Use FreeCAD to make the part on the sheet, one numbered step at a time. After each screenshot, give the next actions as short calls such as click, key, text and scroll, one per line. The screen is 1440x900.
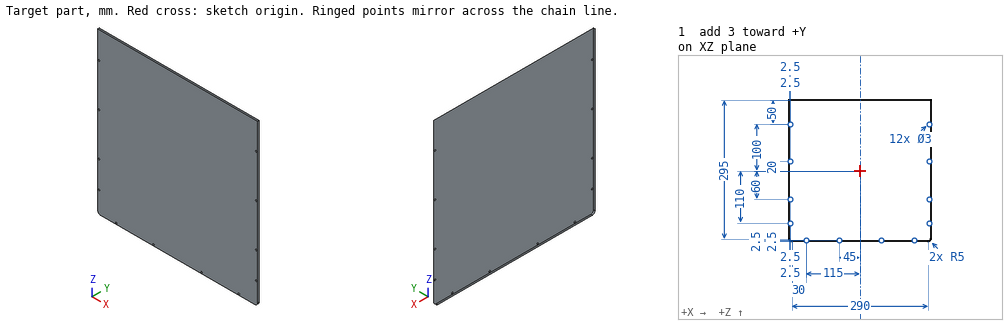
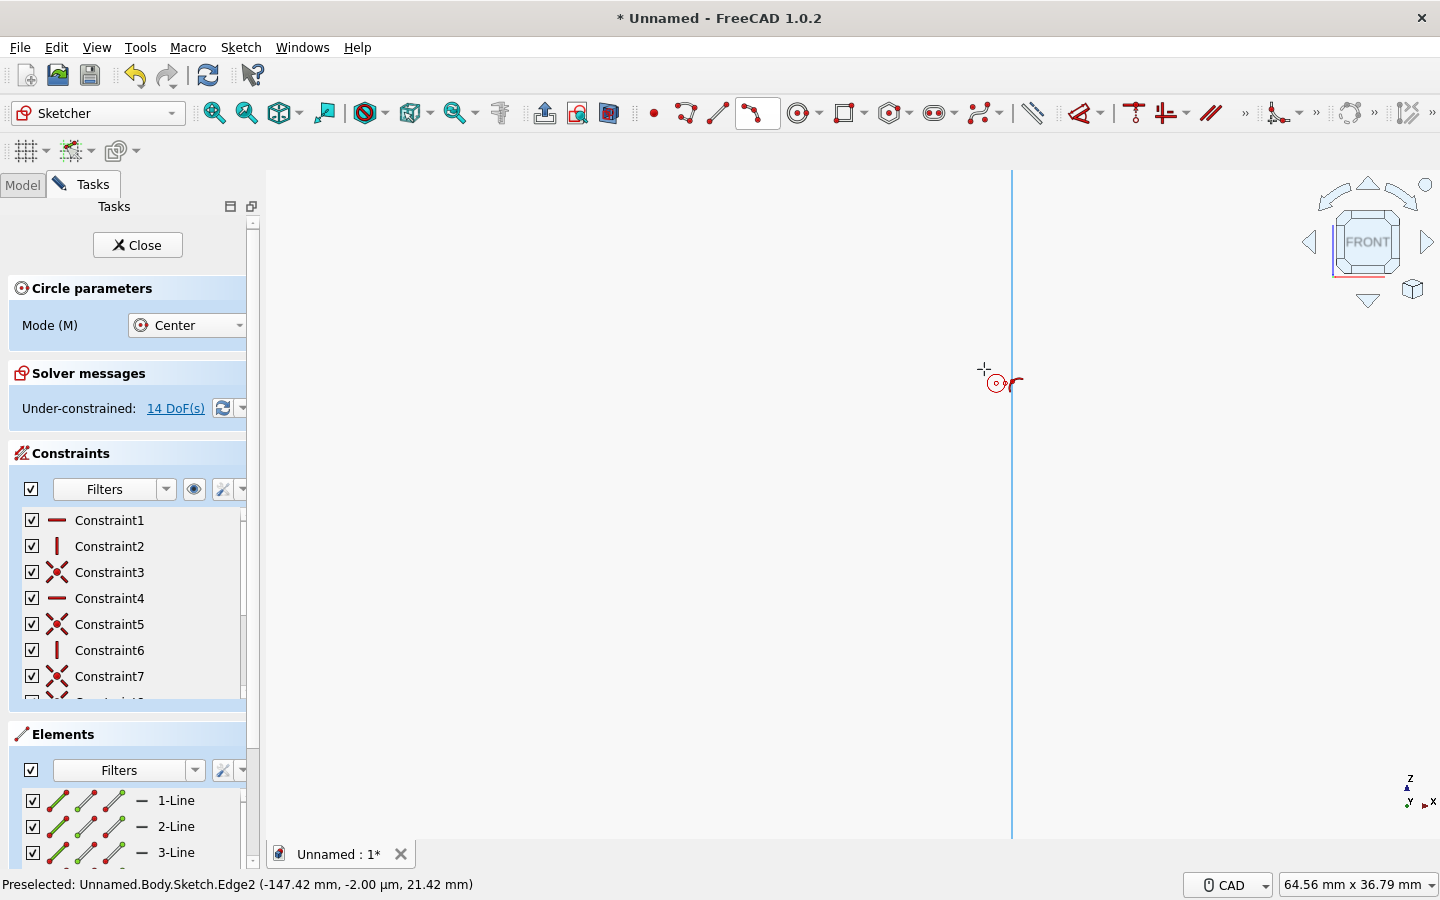
click(971, 371)
move(990, 352)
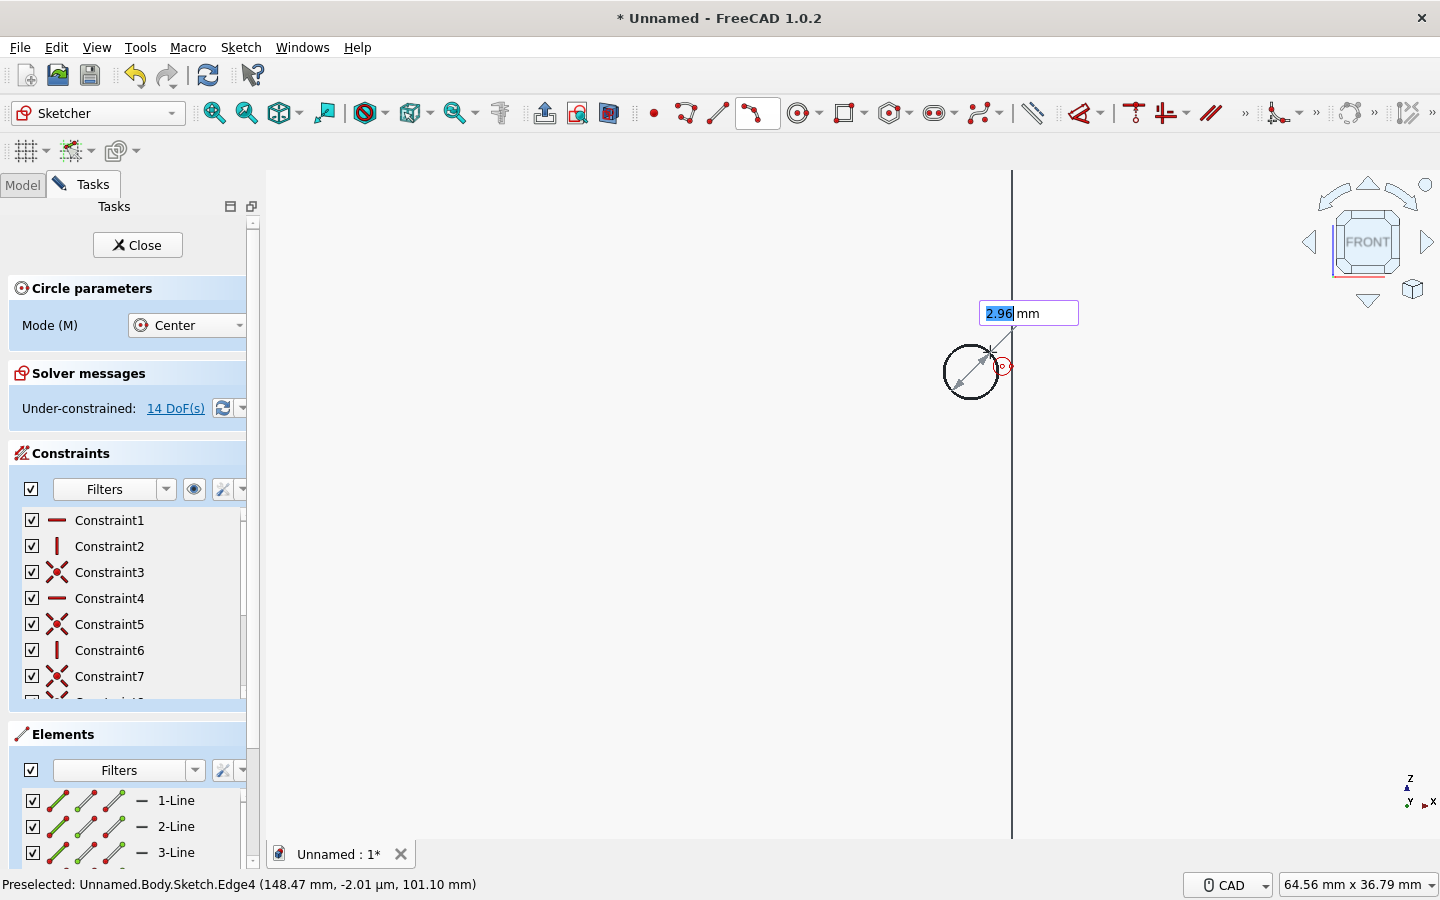
text(3)
key(Return)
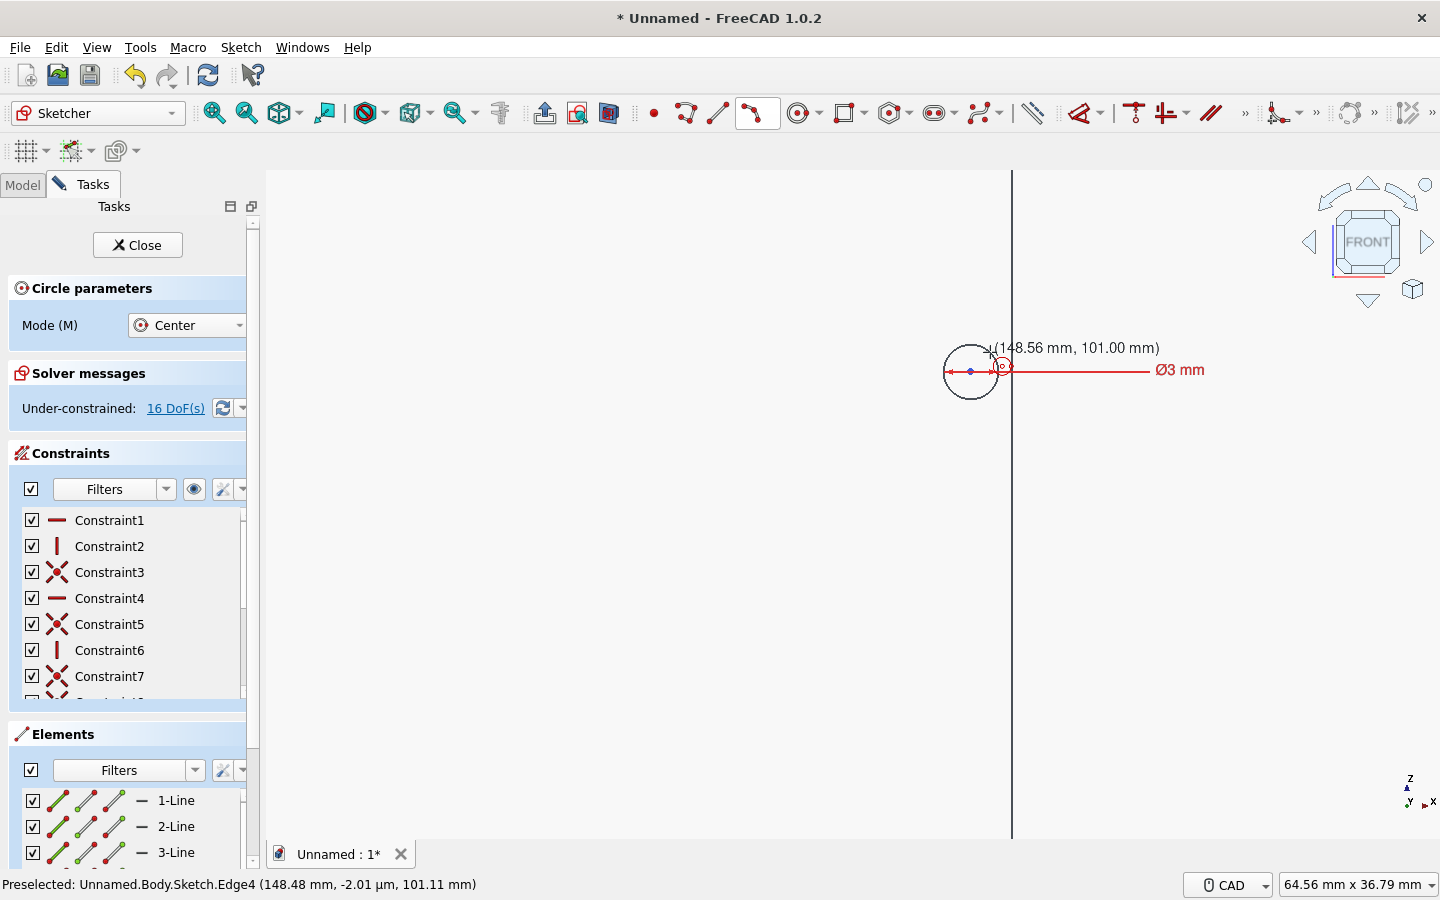
scroll(985, 369, down, 13)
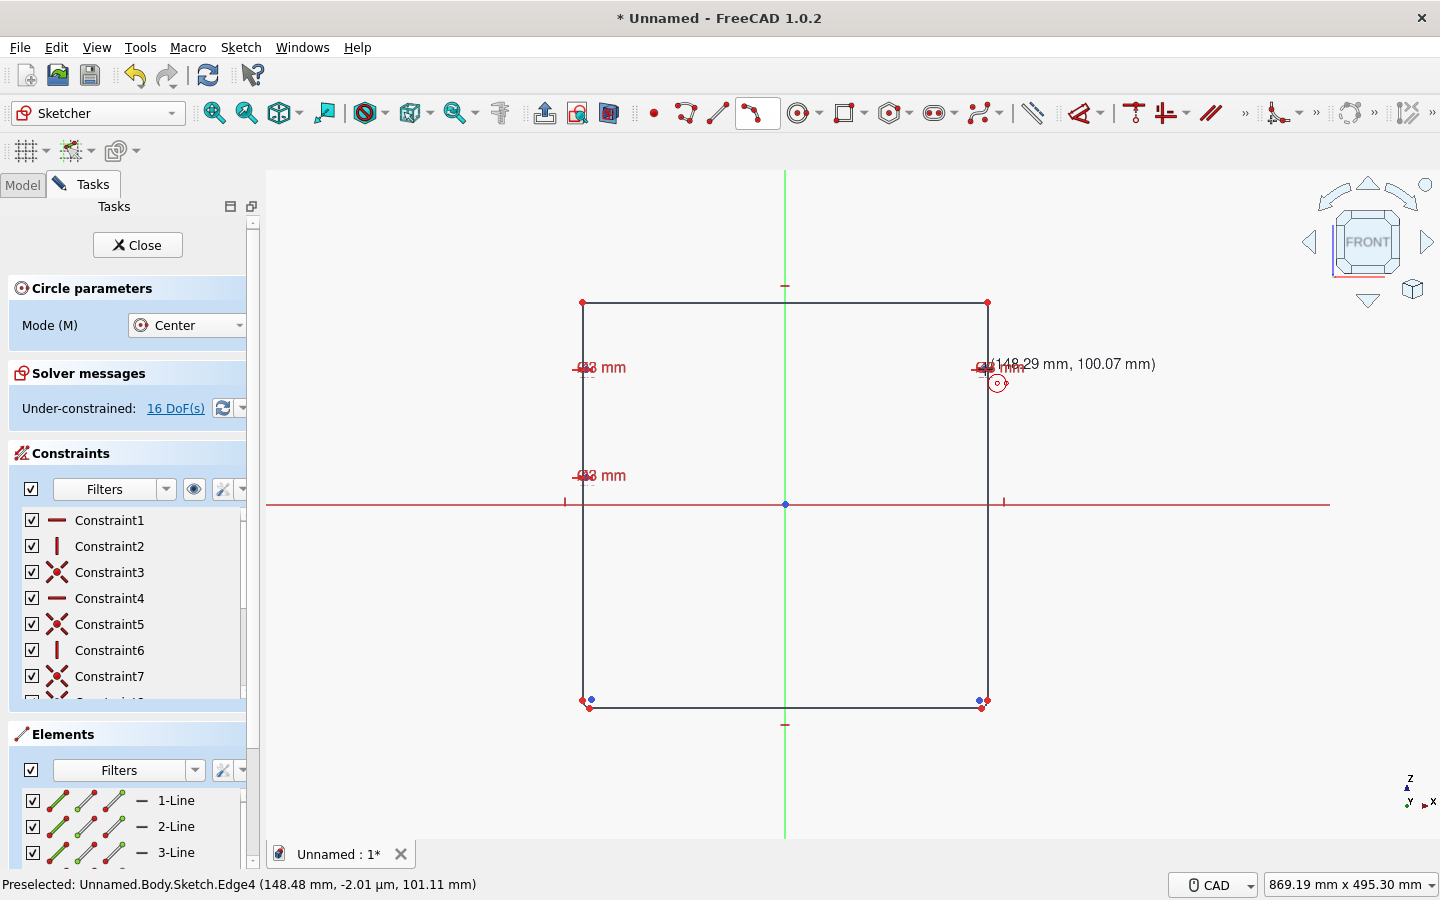
scroll(985, 477, up, 13)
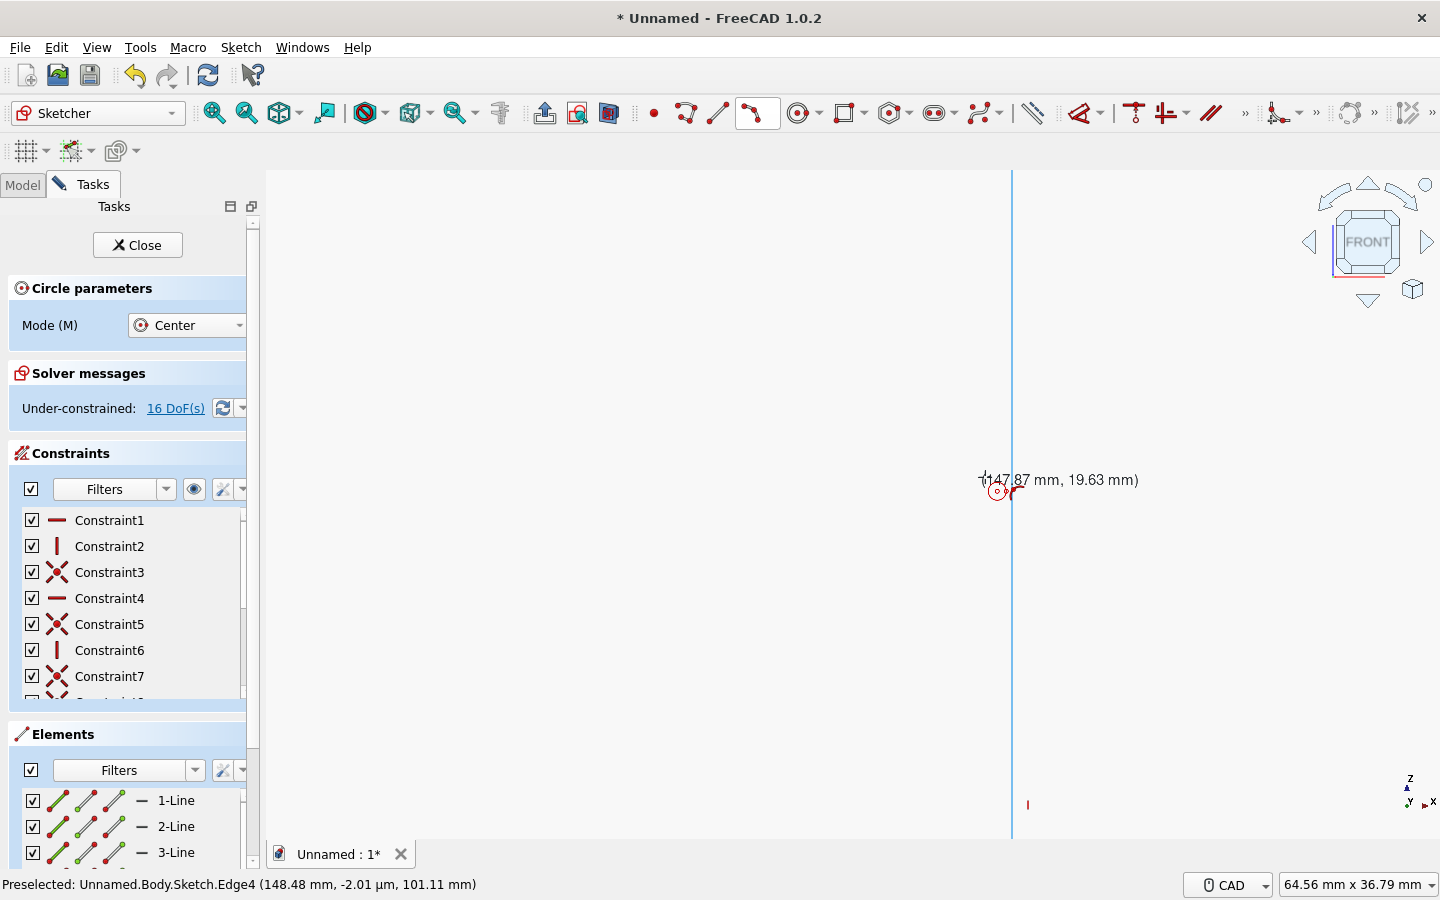
click(971, 478)
move(990, 459)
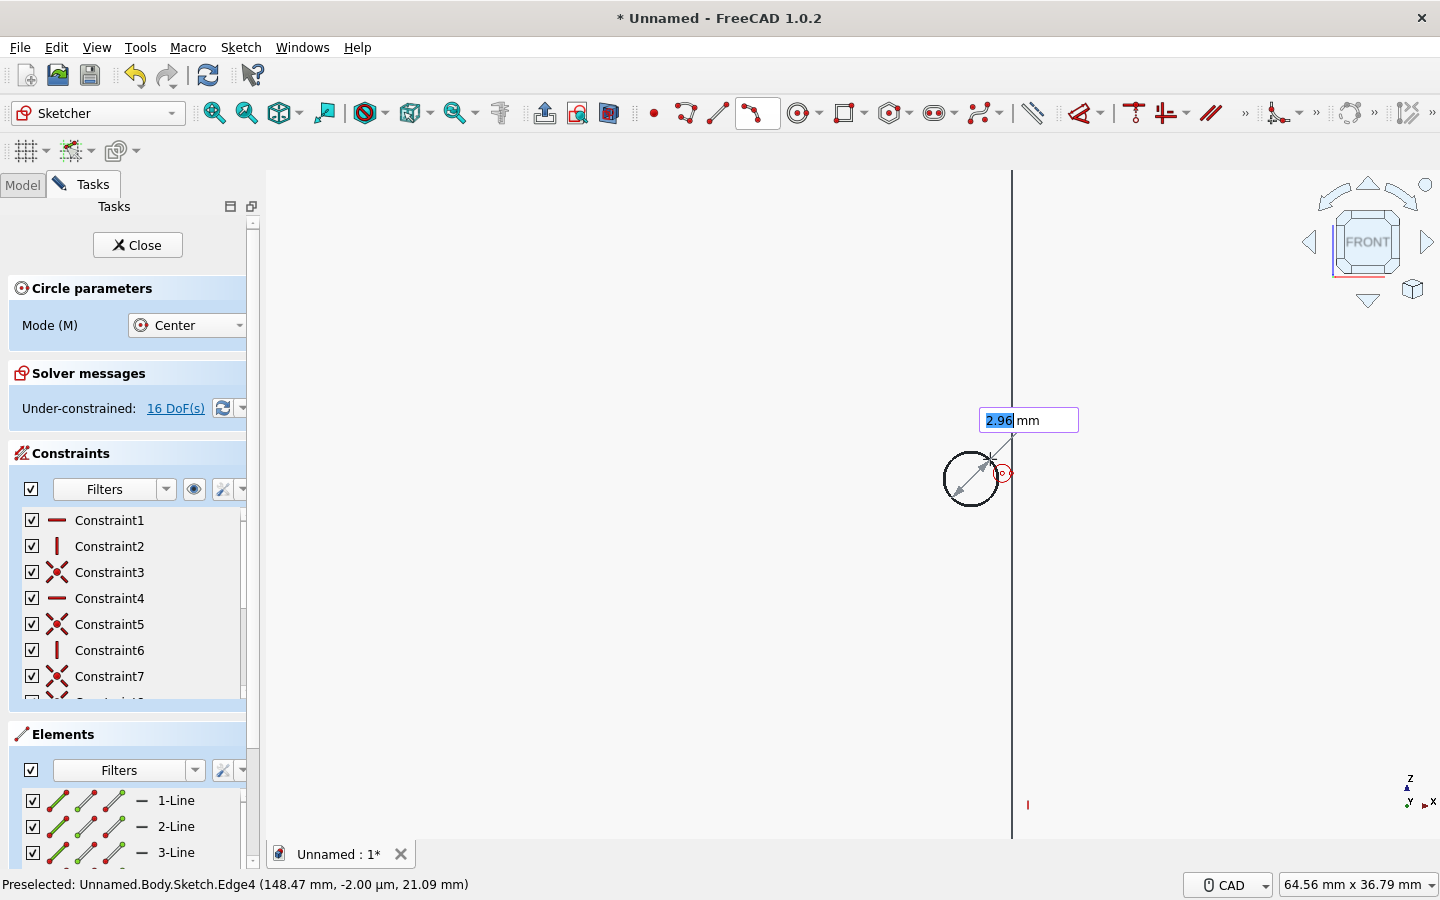
text(3)
key(Return)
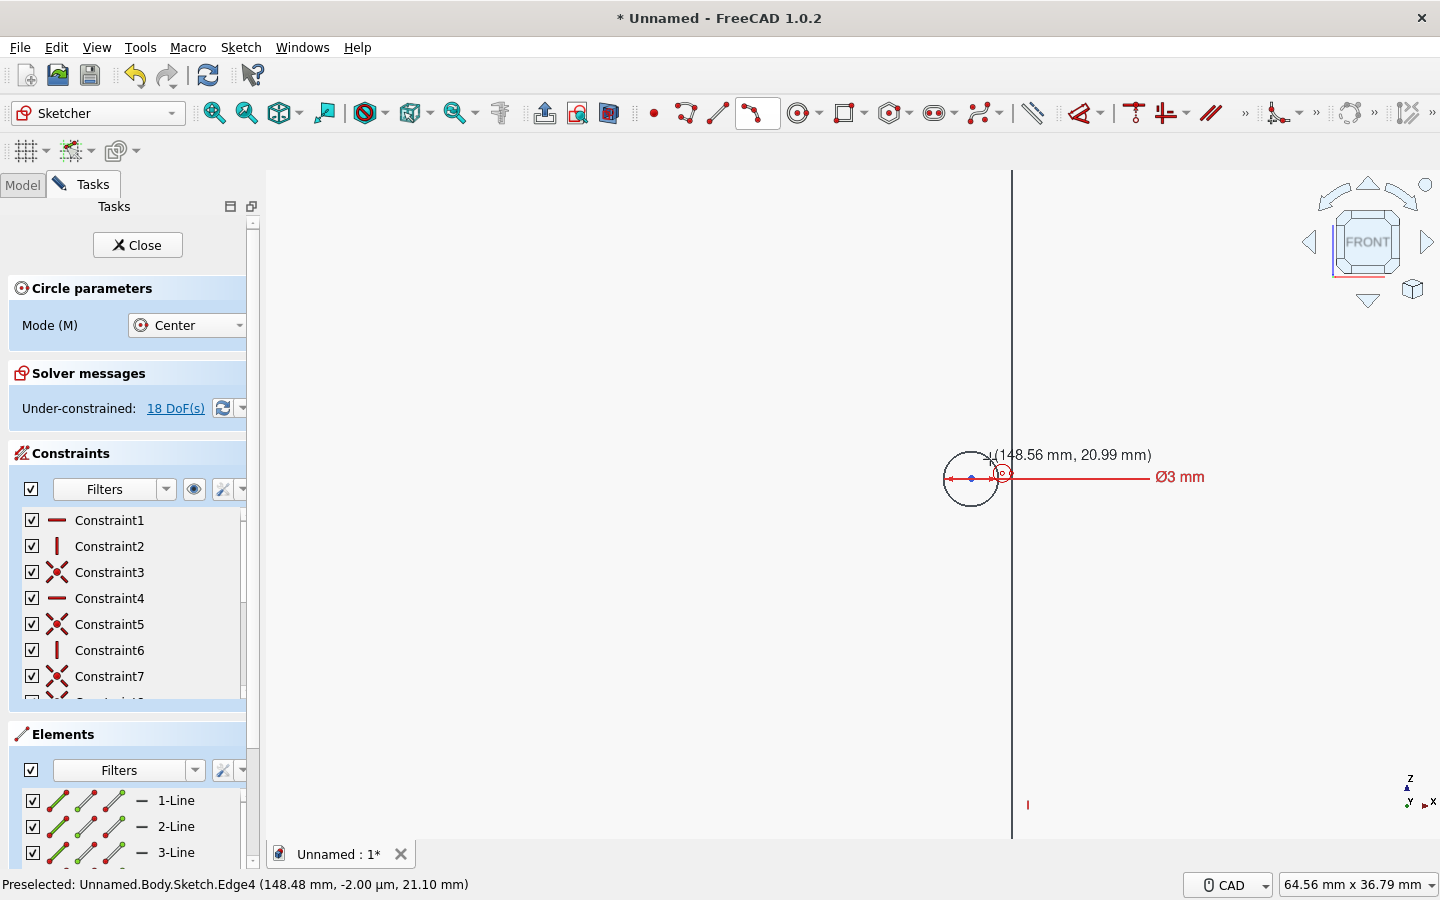
scroll(985, 477, down, 13)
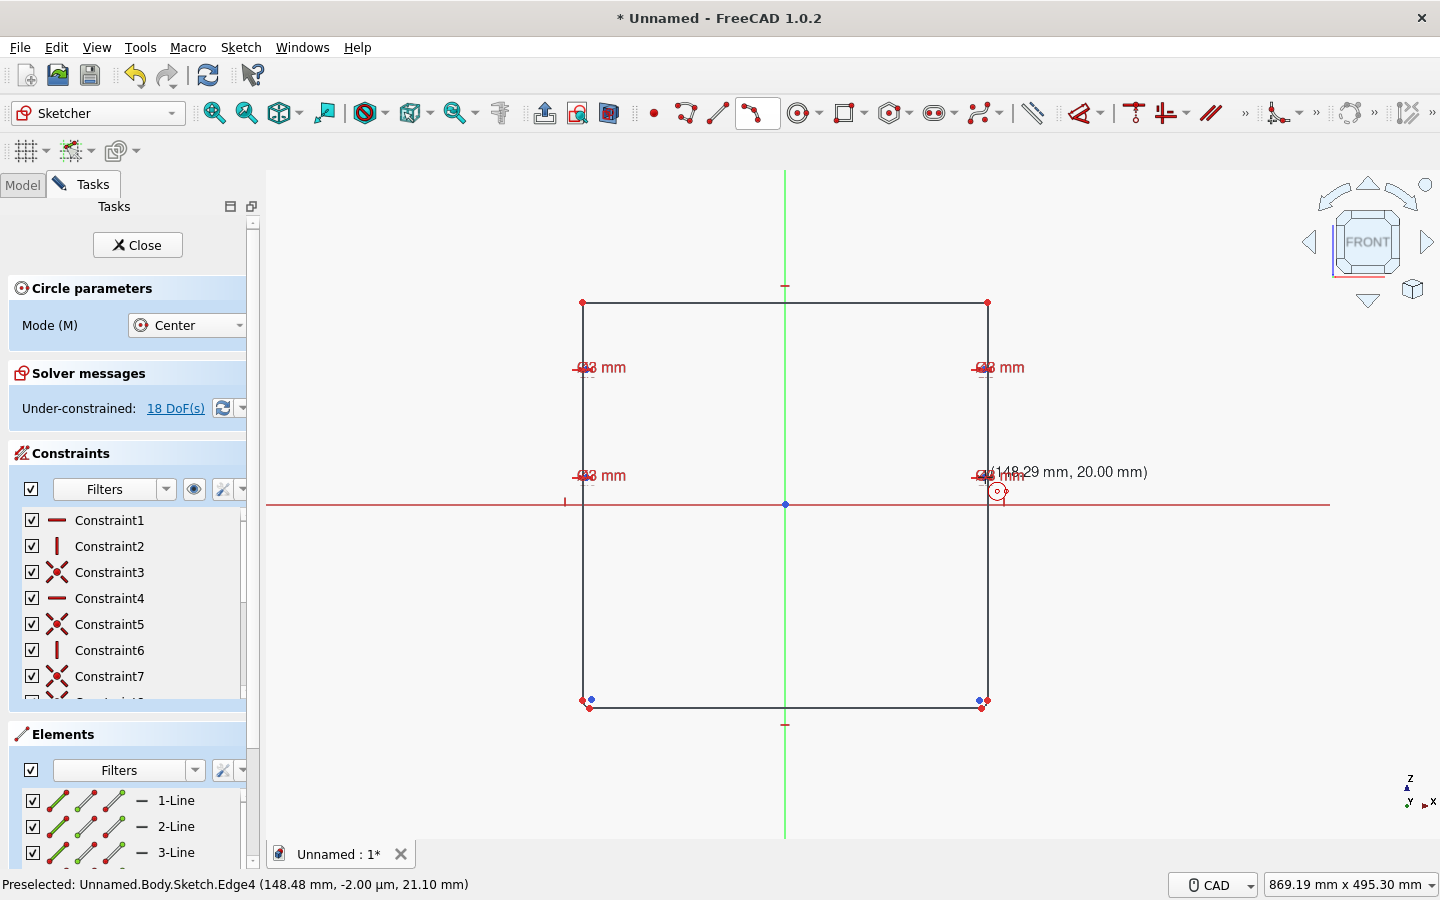
scroll(586, 586, up, 13)